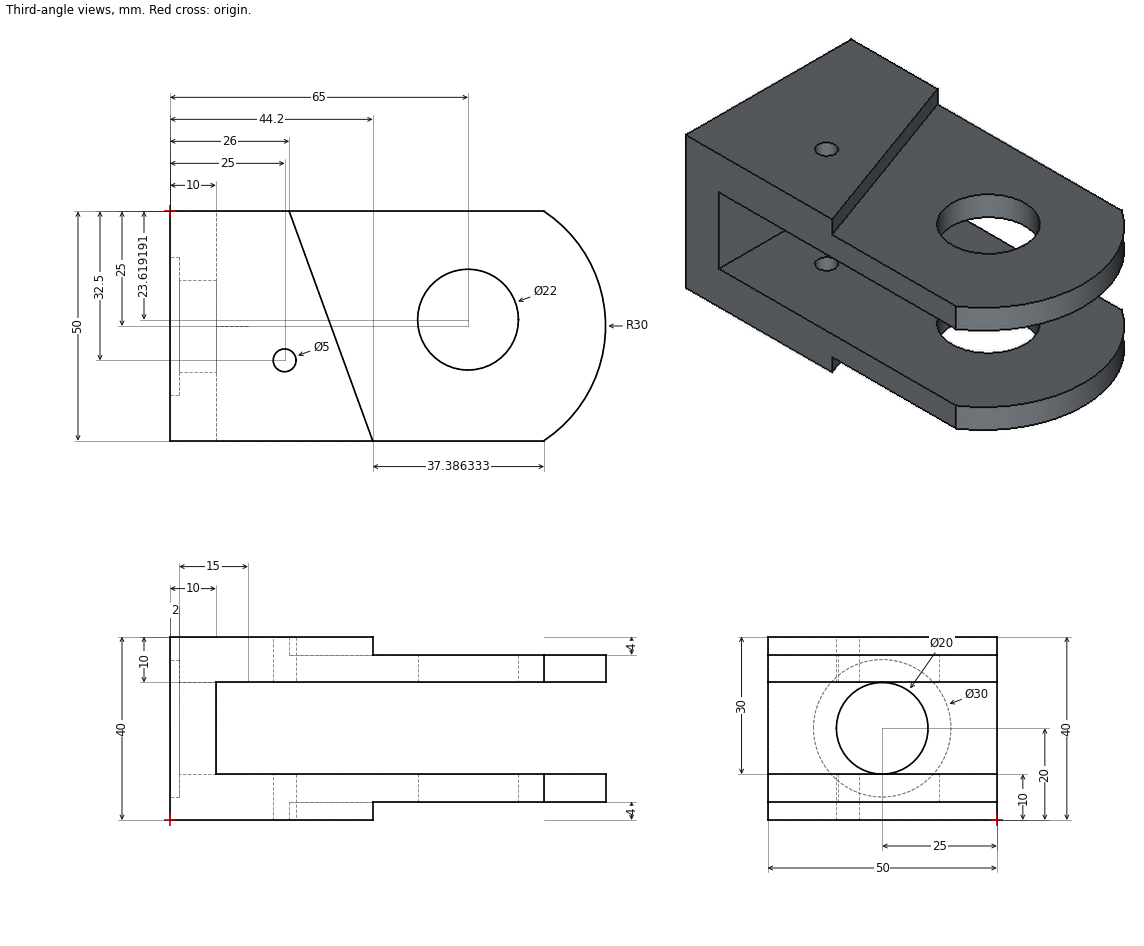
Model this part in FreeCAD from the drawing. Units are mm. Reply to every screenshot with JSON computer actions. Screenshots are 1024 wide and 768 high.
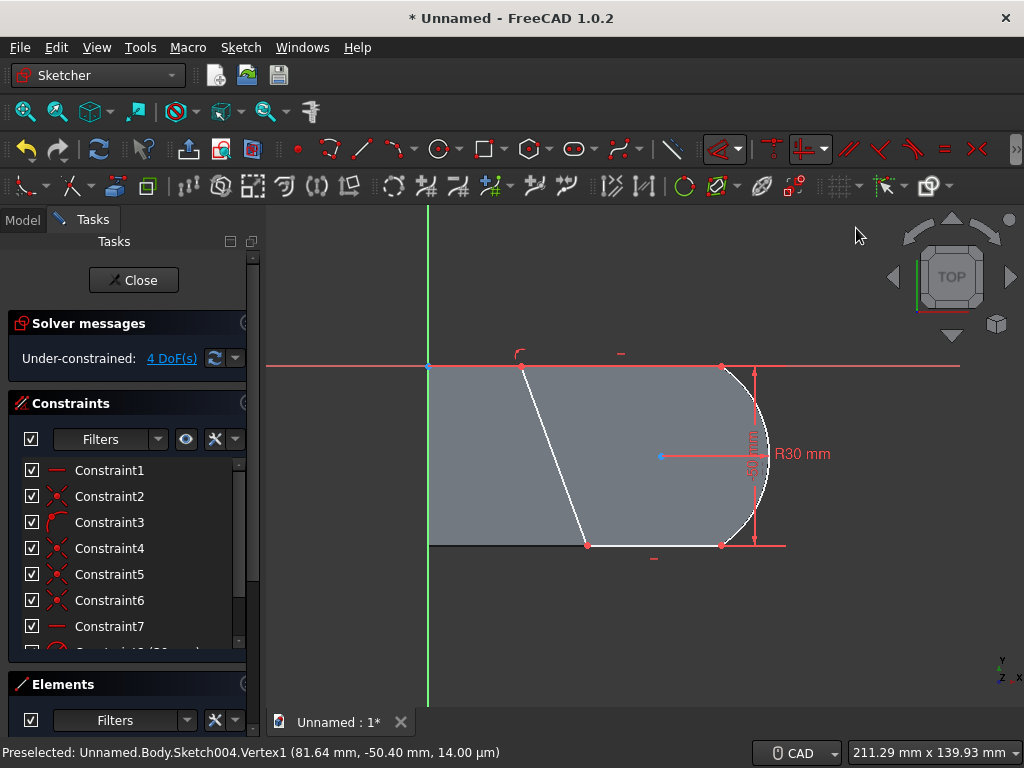
{"action": "left_click", "coordinate": [521, 366]}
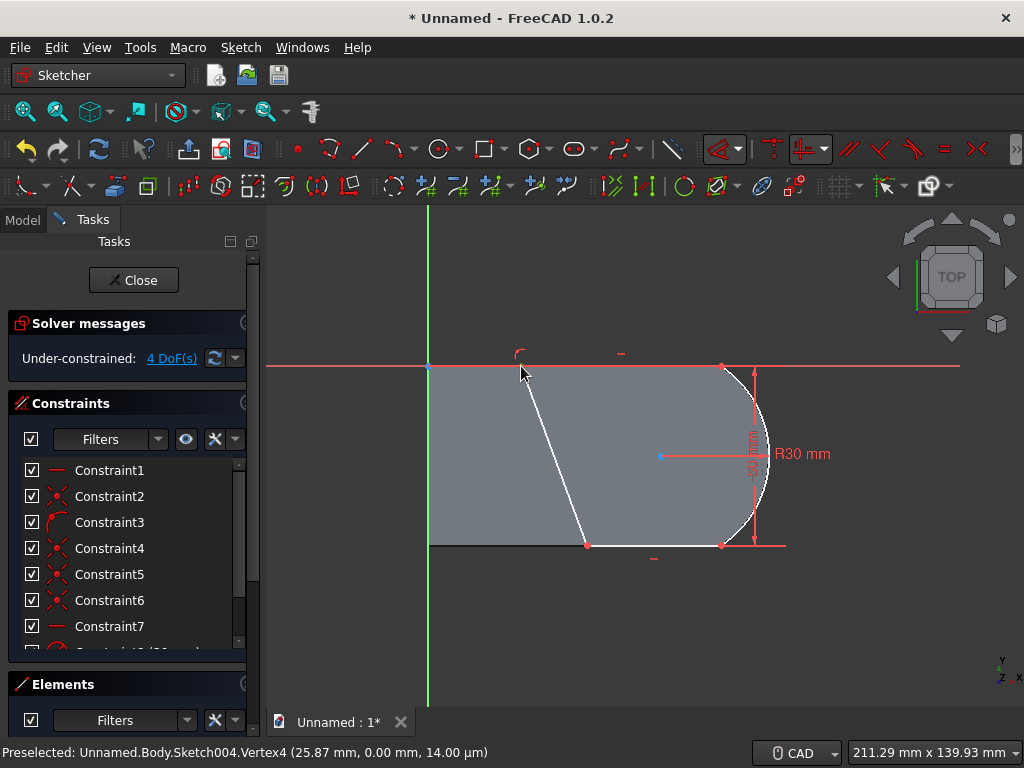
{"action": "left_click", "coordinate": [740, 150]}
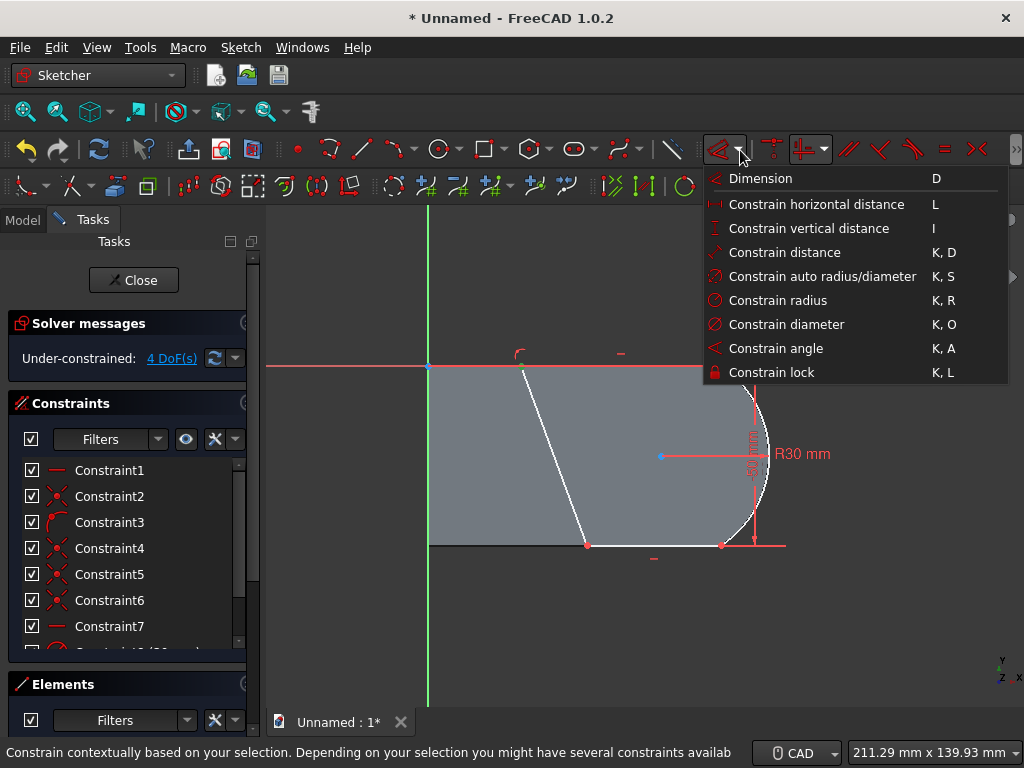
{"action": "left_click", "coordinate": [856, 204]}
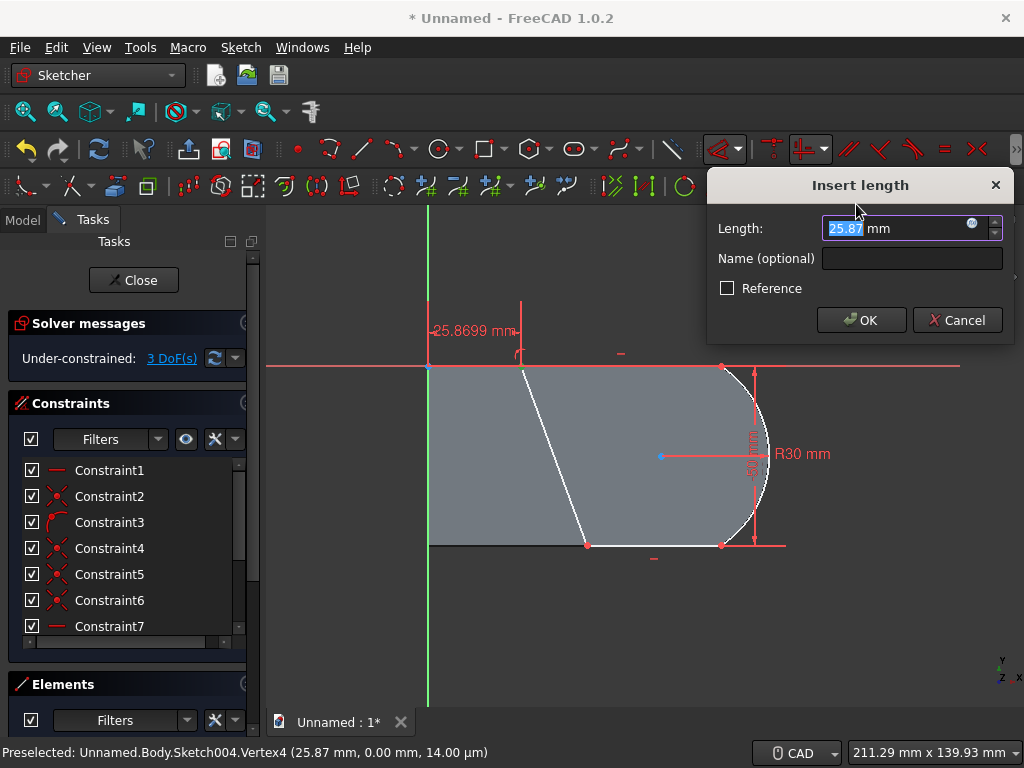
{"action": "type", "text": "26"}
{"action": "key", "text": "Return"}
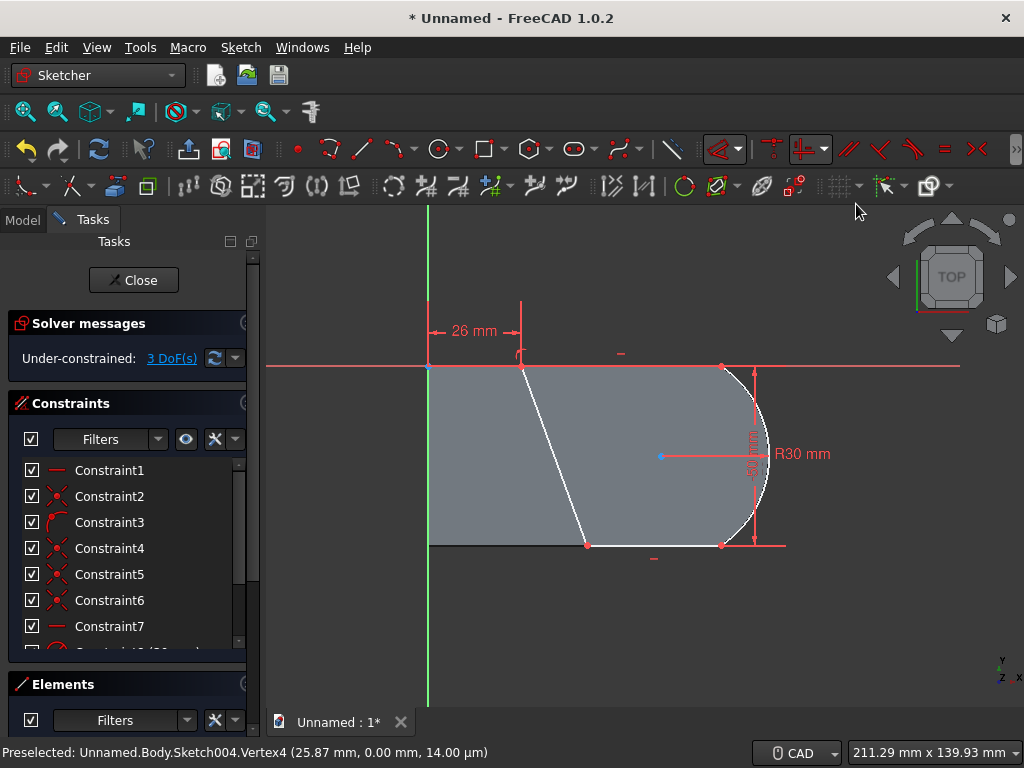
{"action": "left_click", "coordinate": [662, 456]}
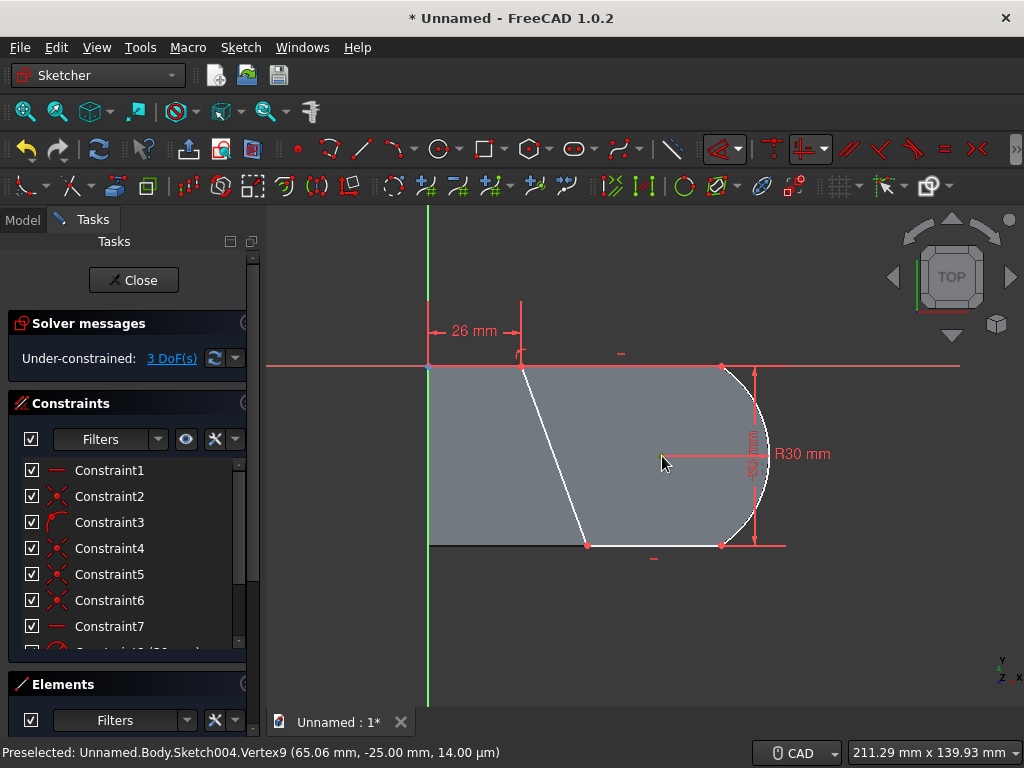
{"action": "left_click", "coordinate": [740, 150]}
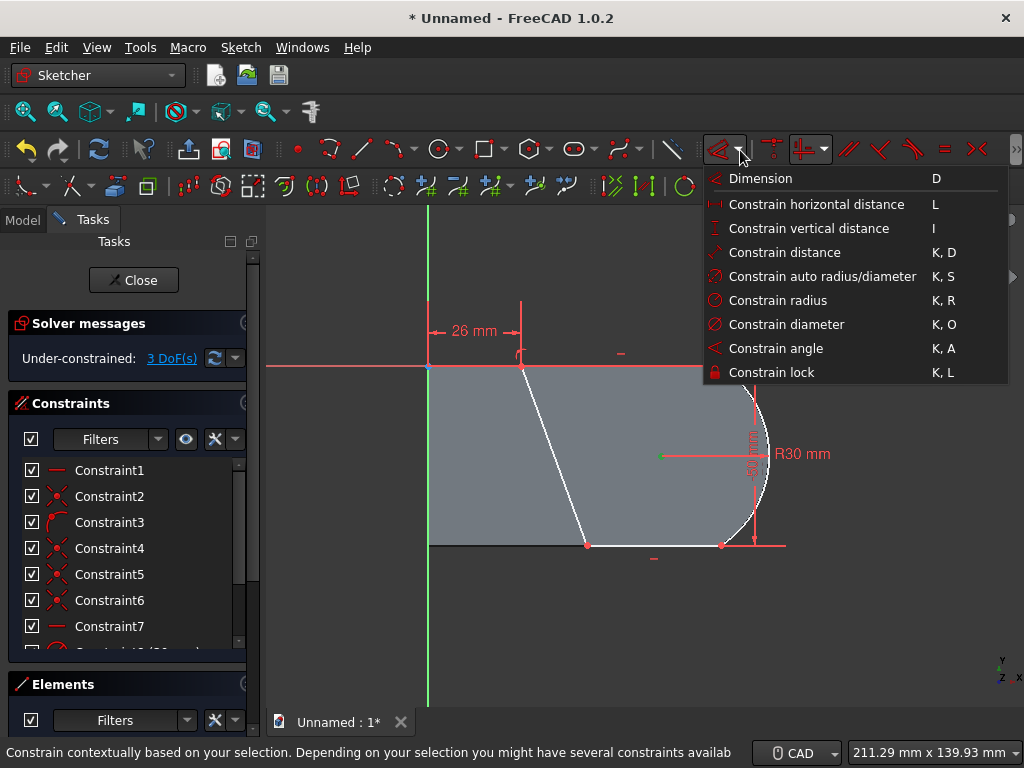
{"action": "left_click", "coordinate": [856, 204]}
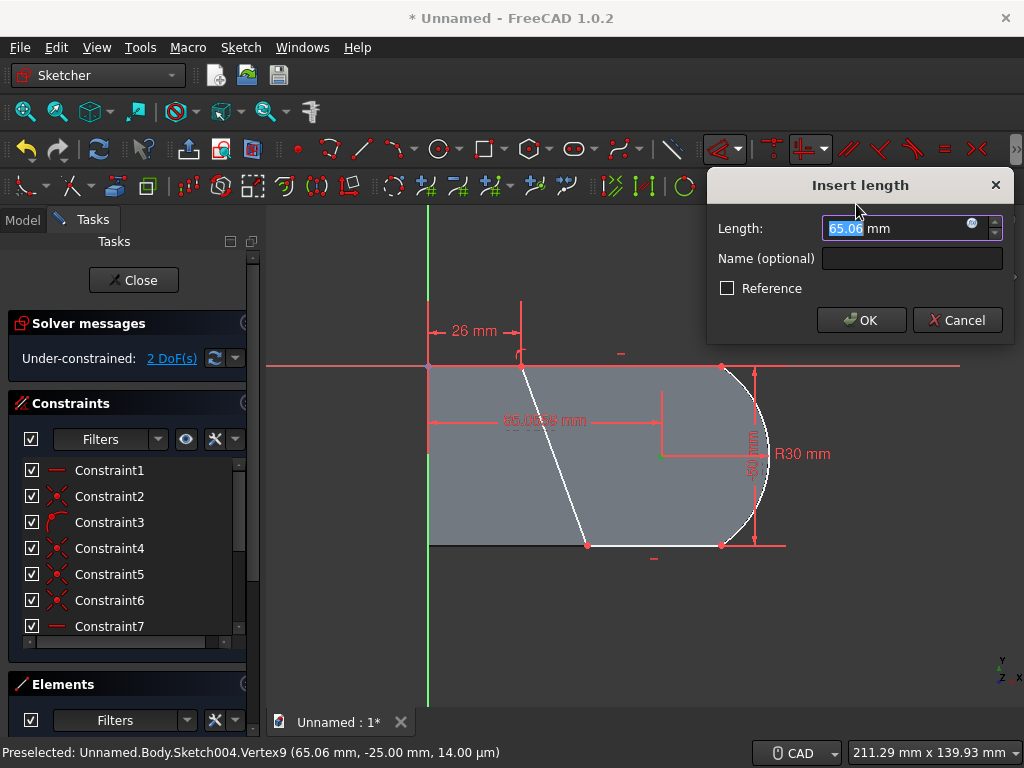
{"action": "type", "text": "65"}
{"action": "key", "text": "Return"}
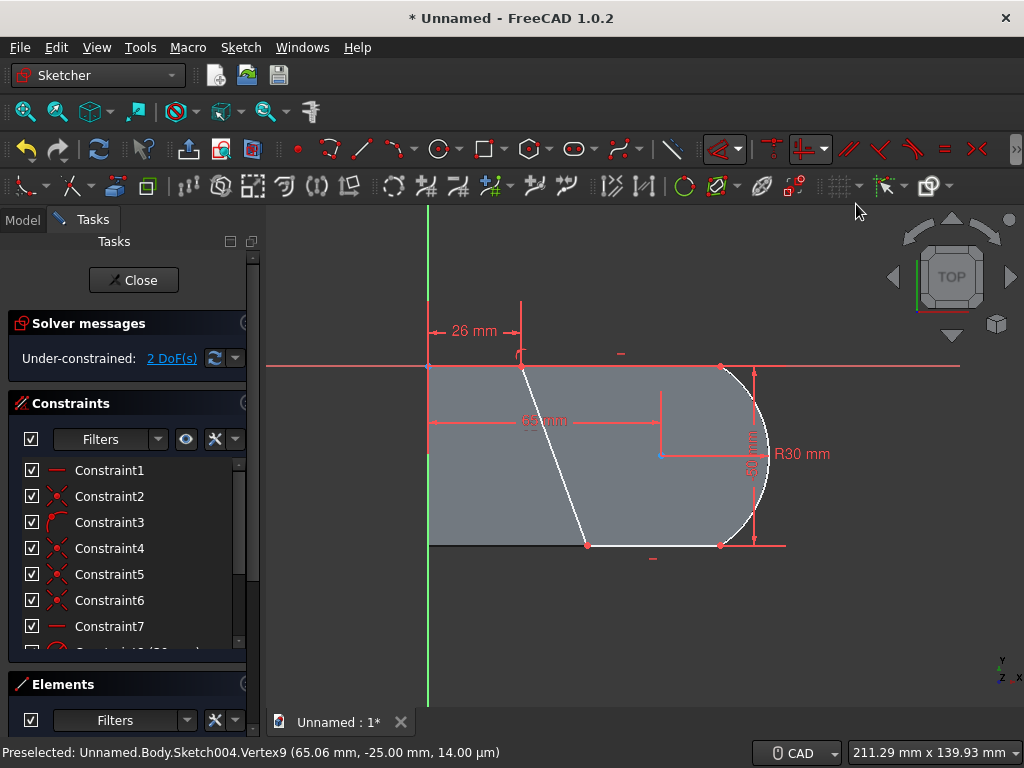
{"action": "left_click", "coordinate": [661, 456]}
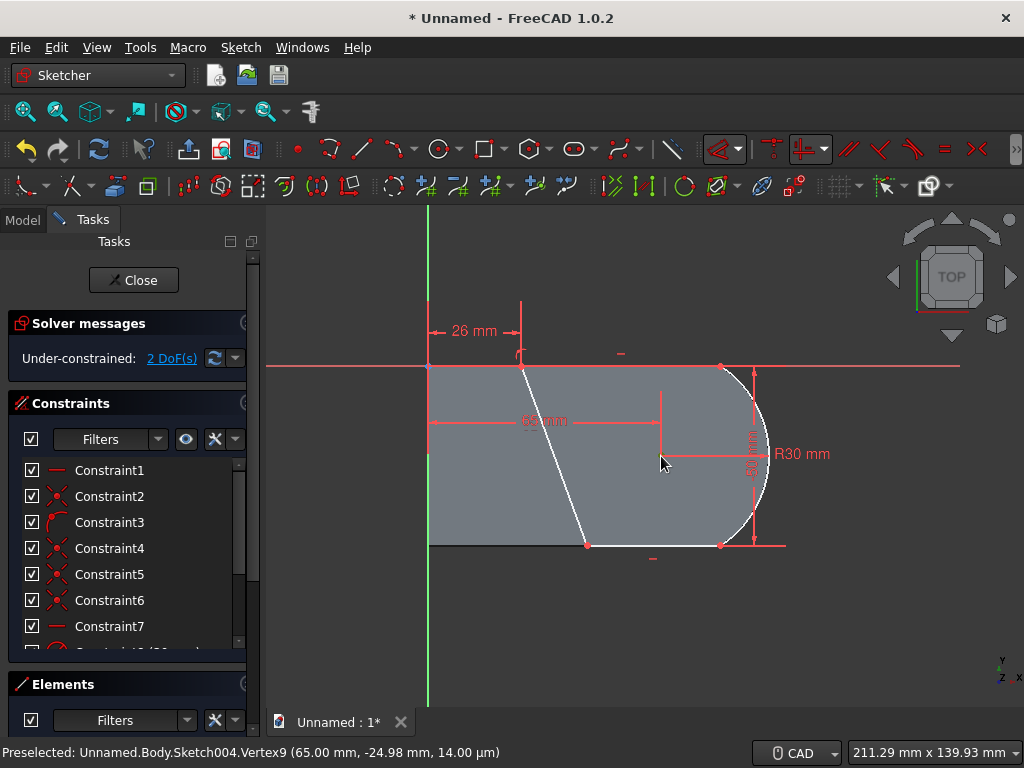
{"action": "left_click", "coordinate": [740, 150]}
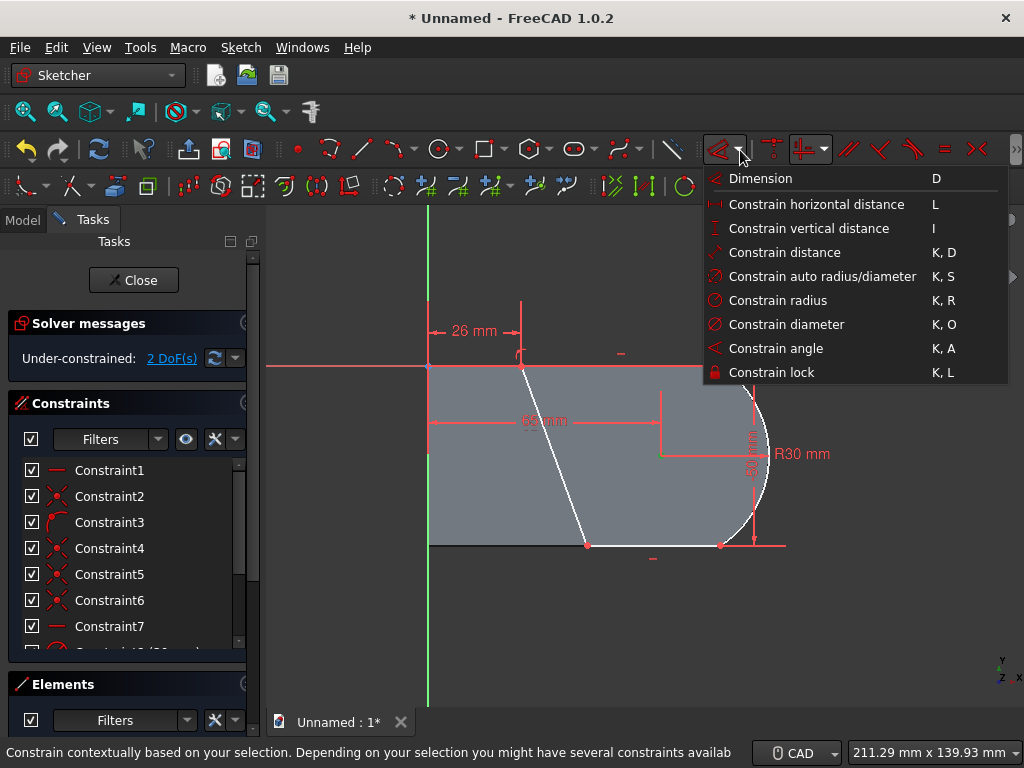
{"action": "left_click", "coordinate": [856, 228]}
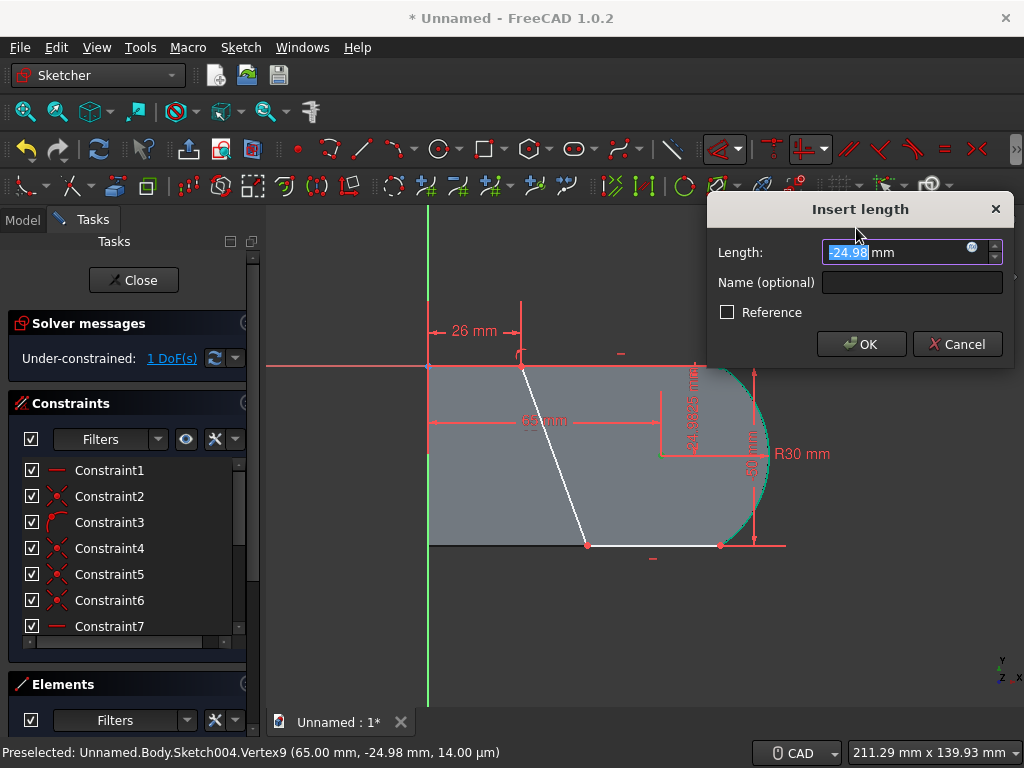
{"action": "type", "text": "-25"}
{"action": "key", "text": "Return"}